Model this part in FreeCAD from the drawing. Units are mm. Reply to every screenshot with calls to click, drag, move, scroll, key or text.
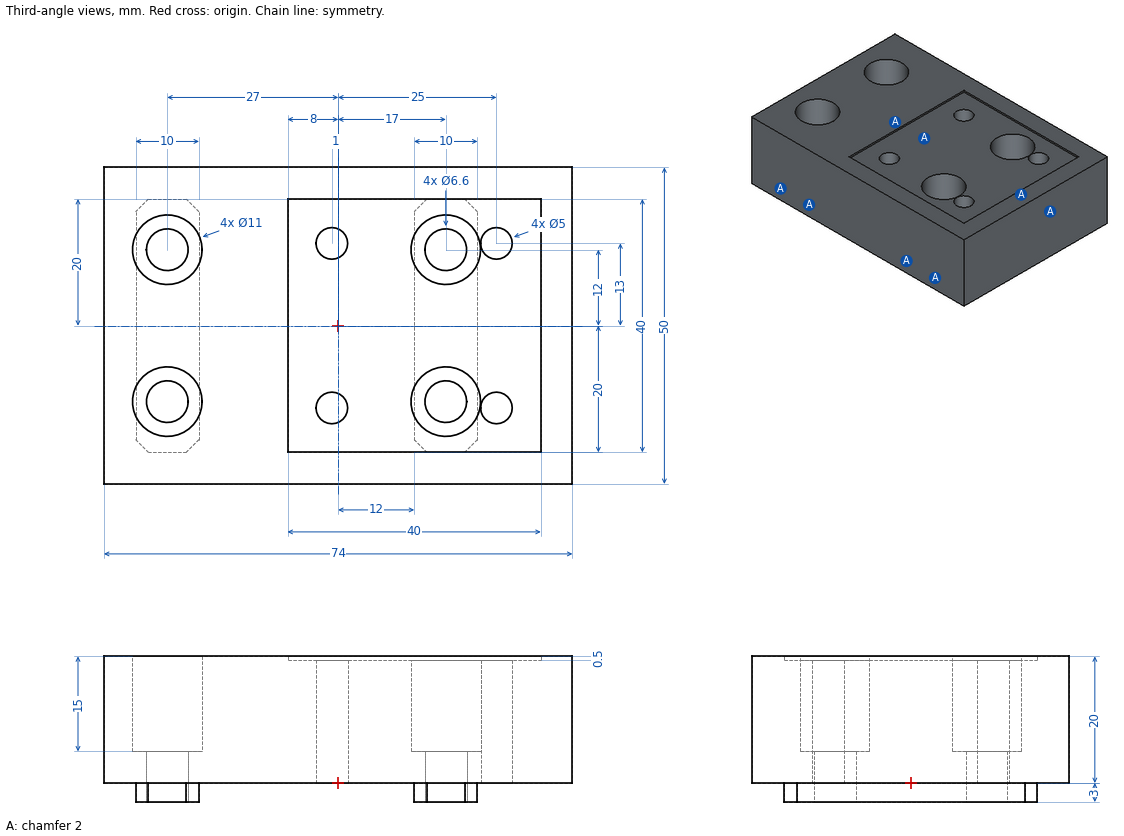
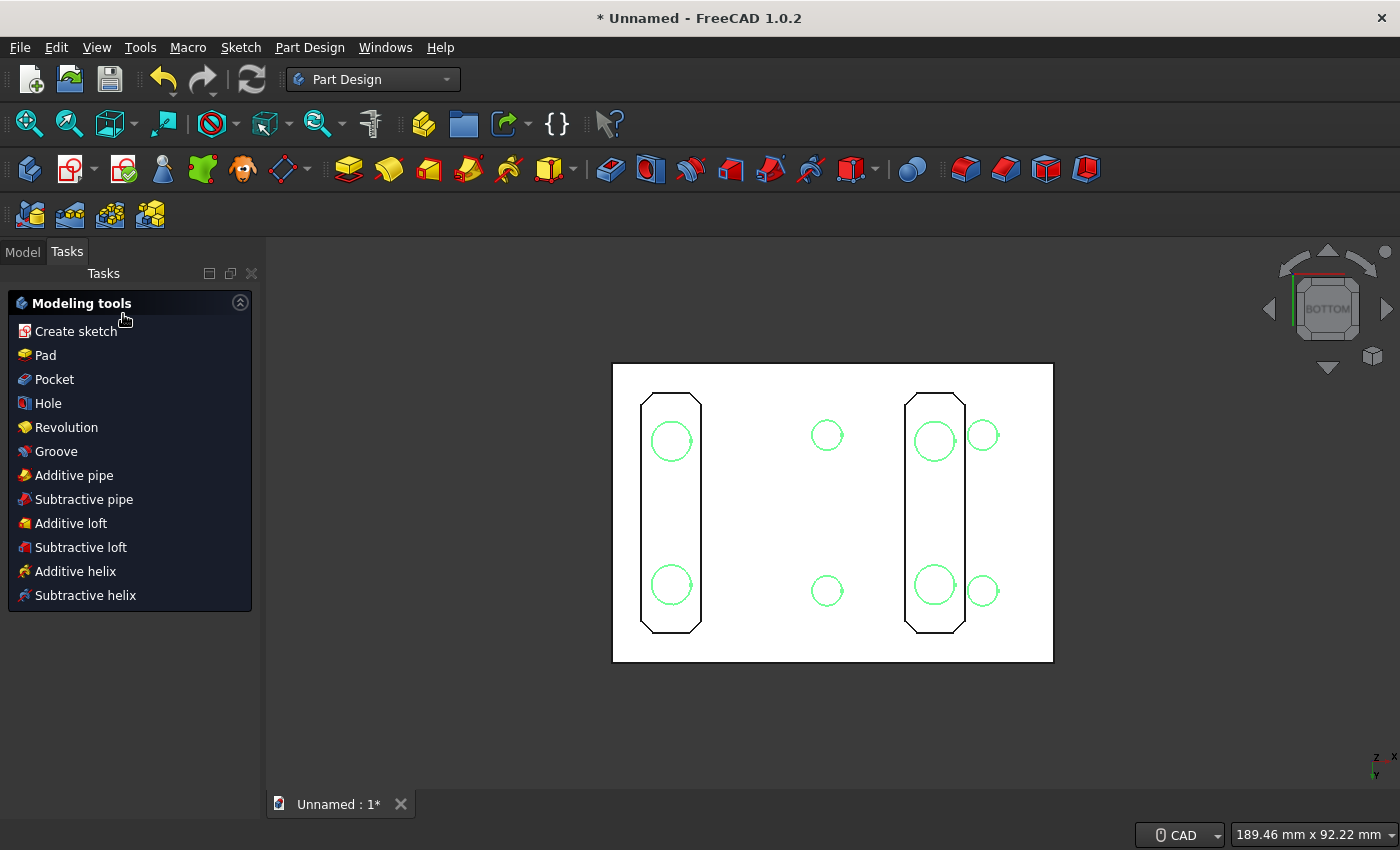
click(612, 170)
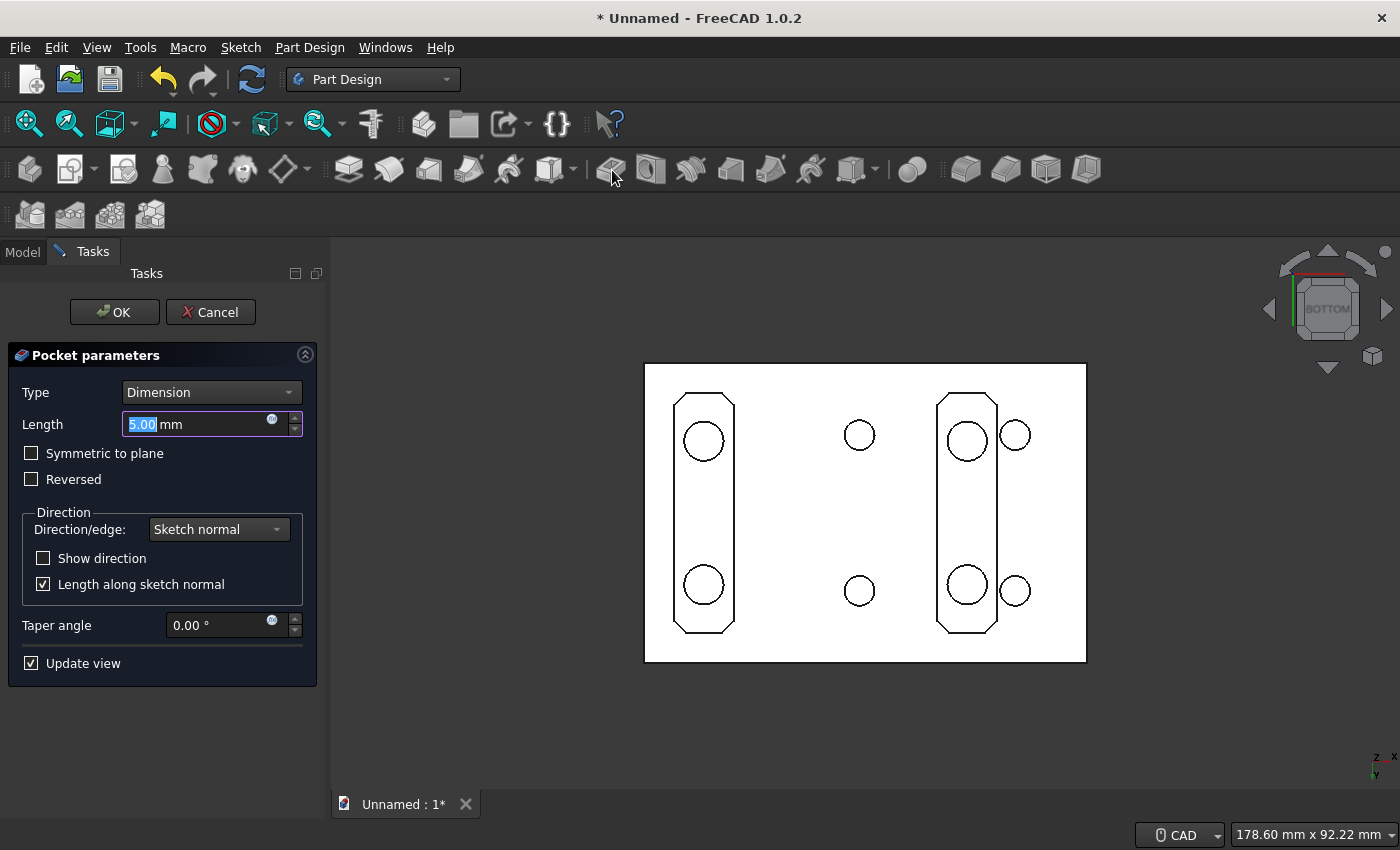
click(212, 392)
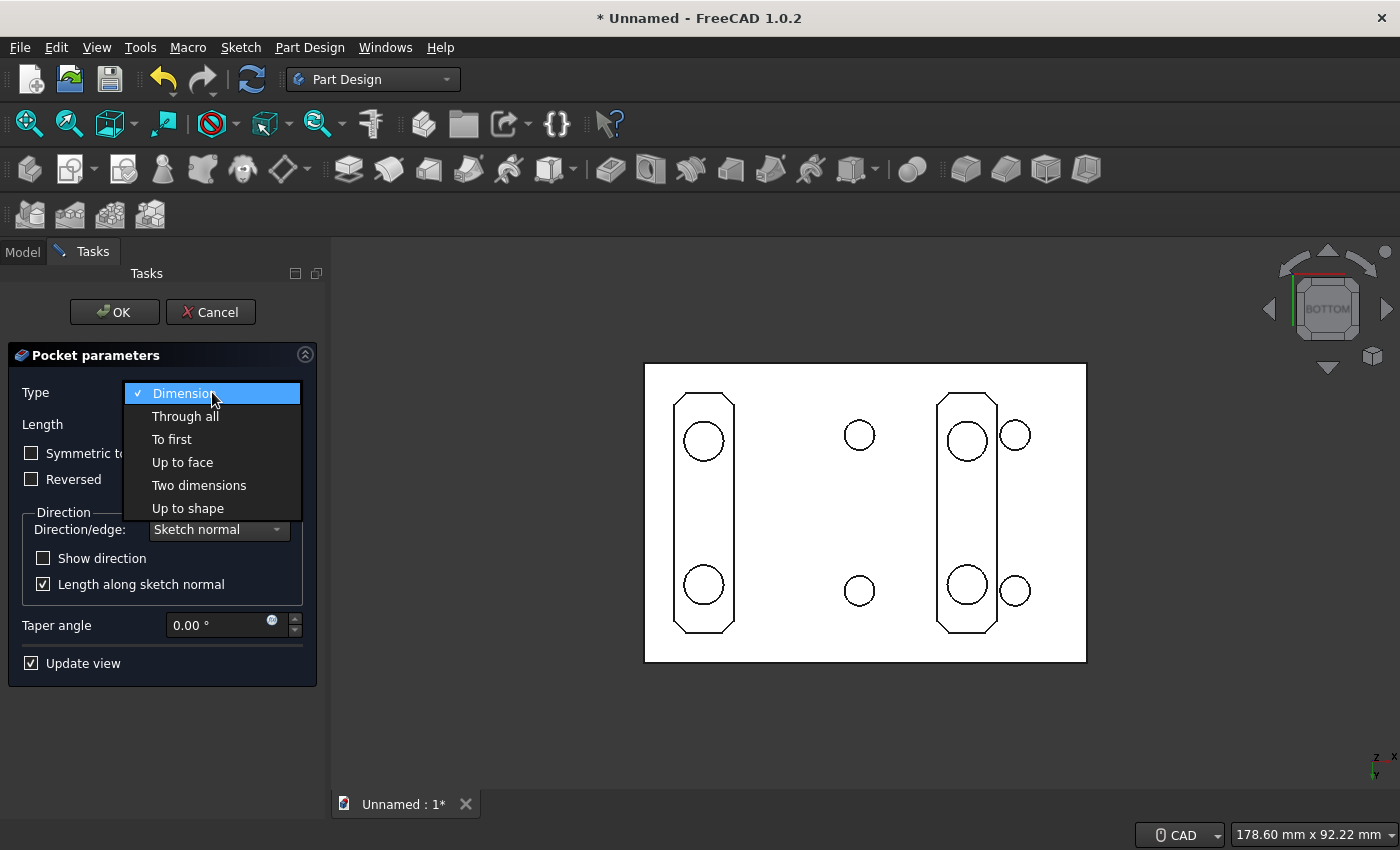
click(212, 416)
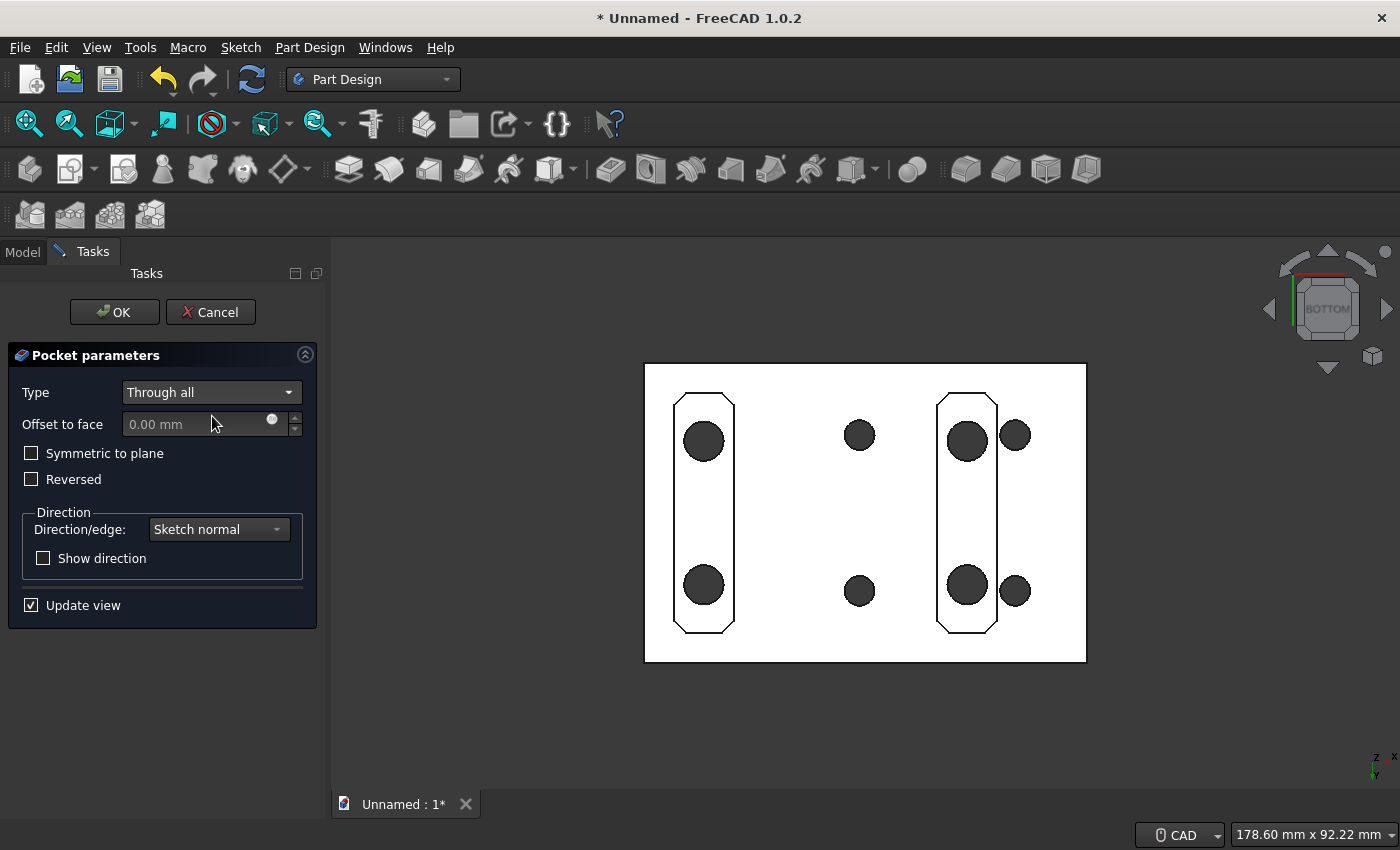
click(115, 312)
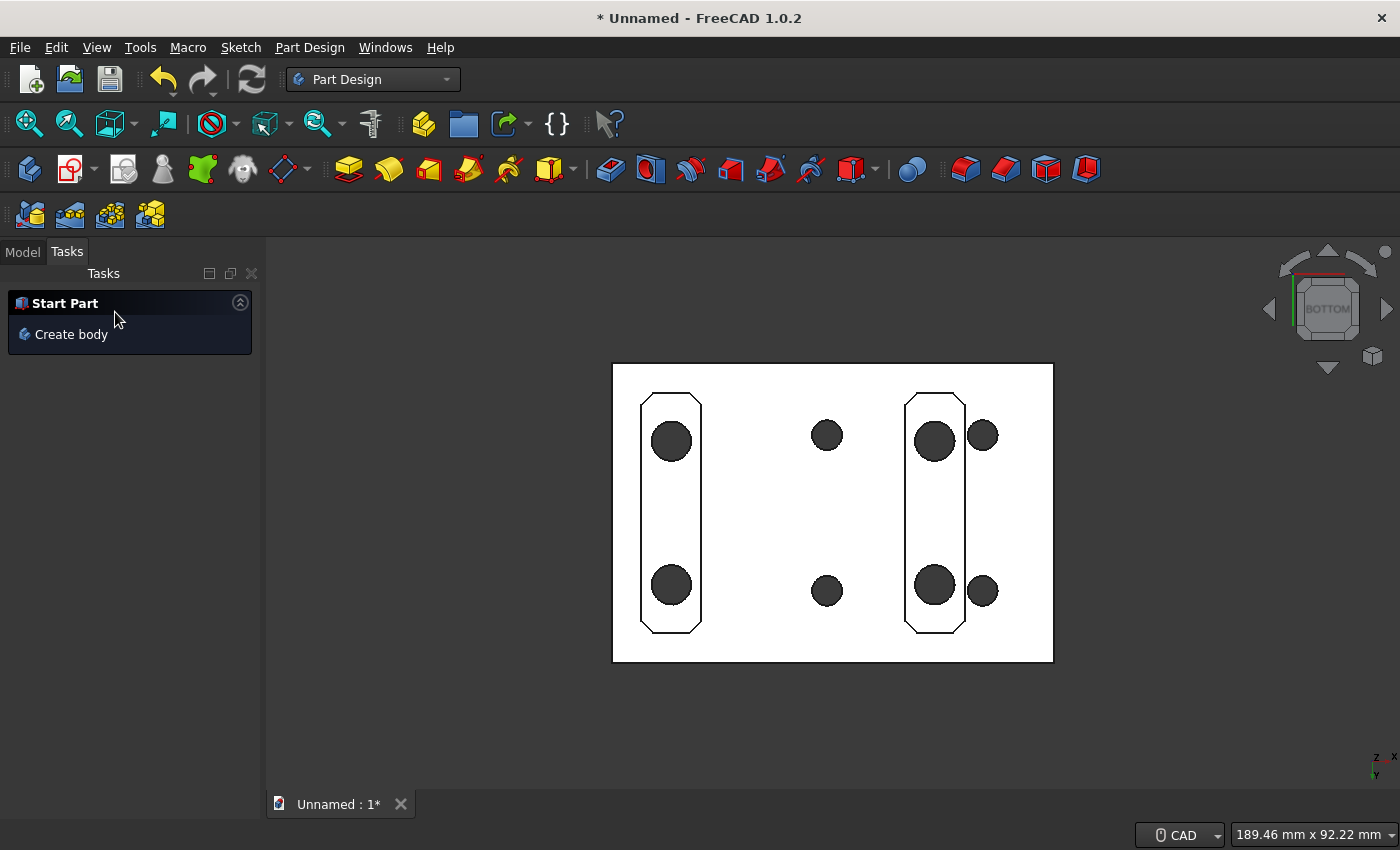
key(0)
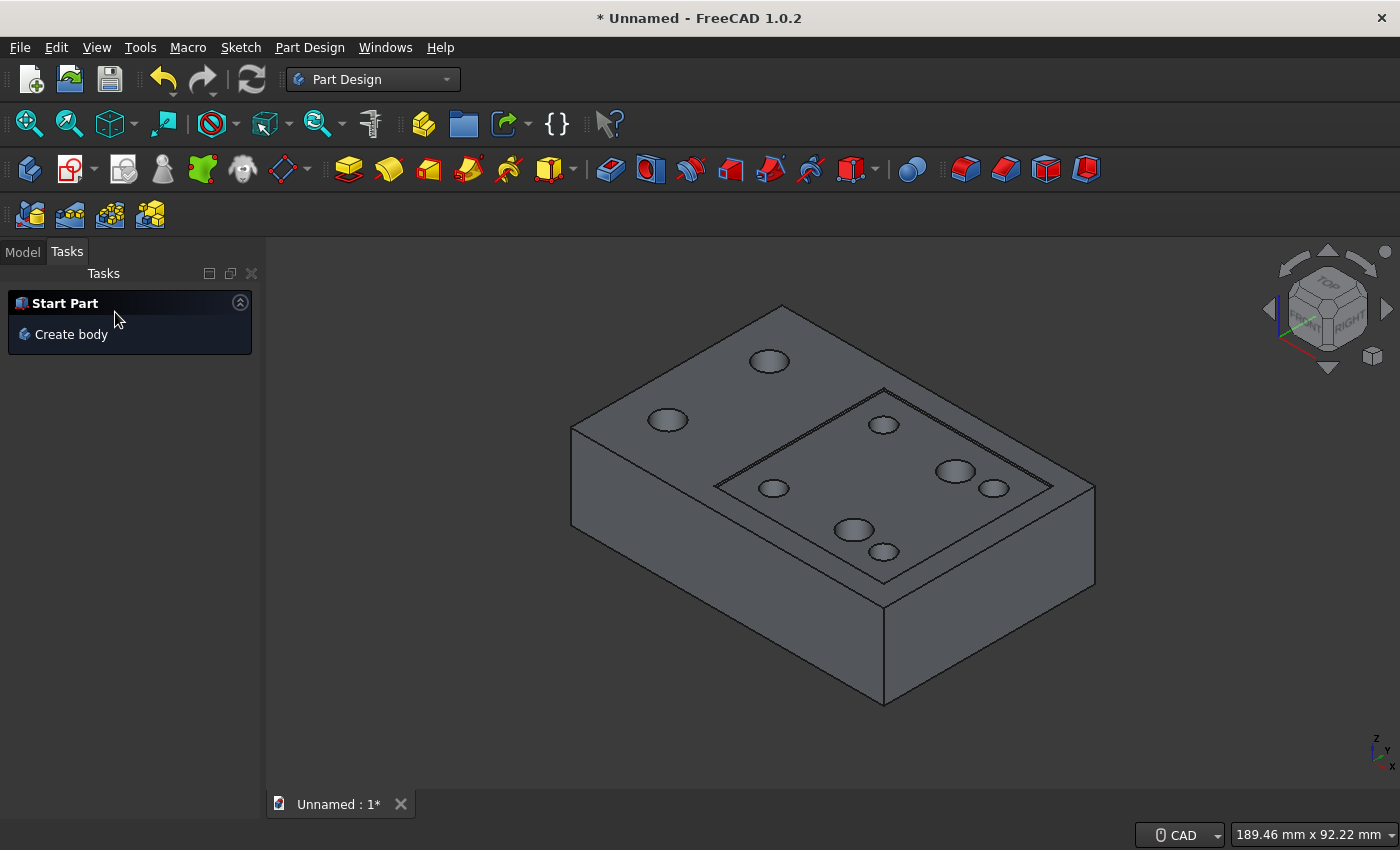
click(744, 404)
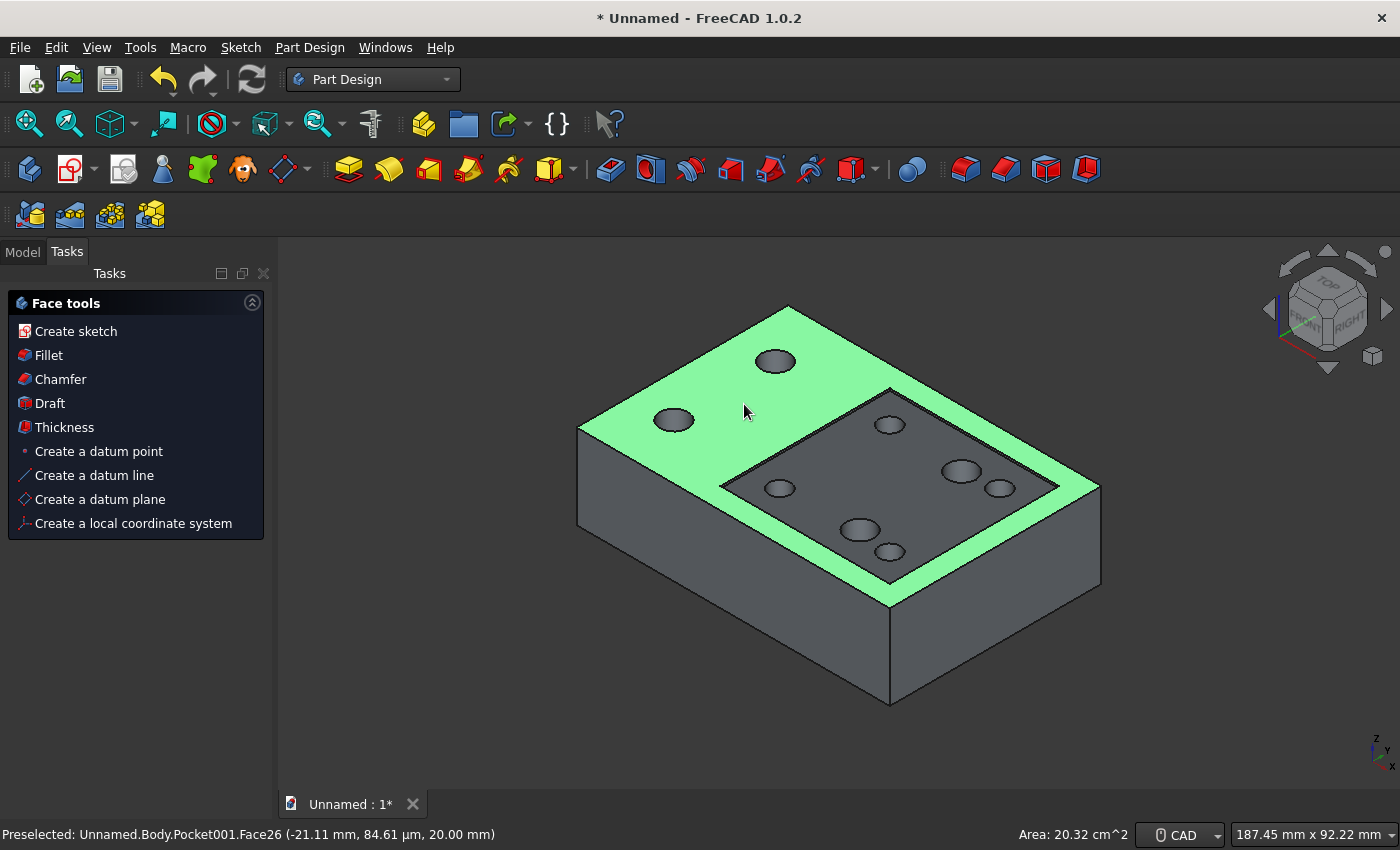
click(70, 170)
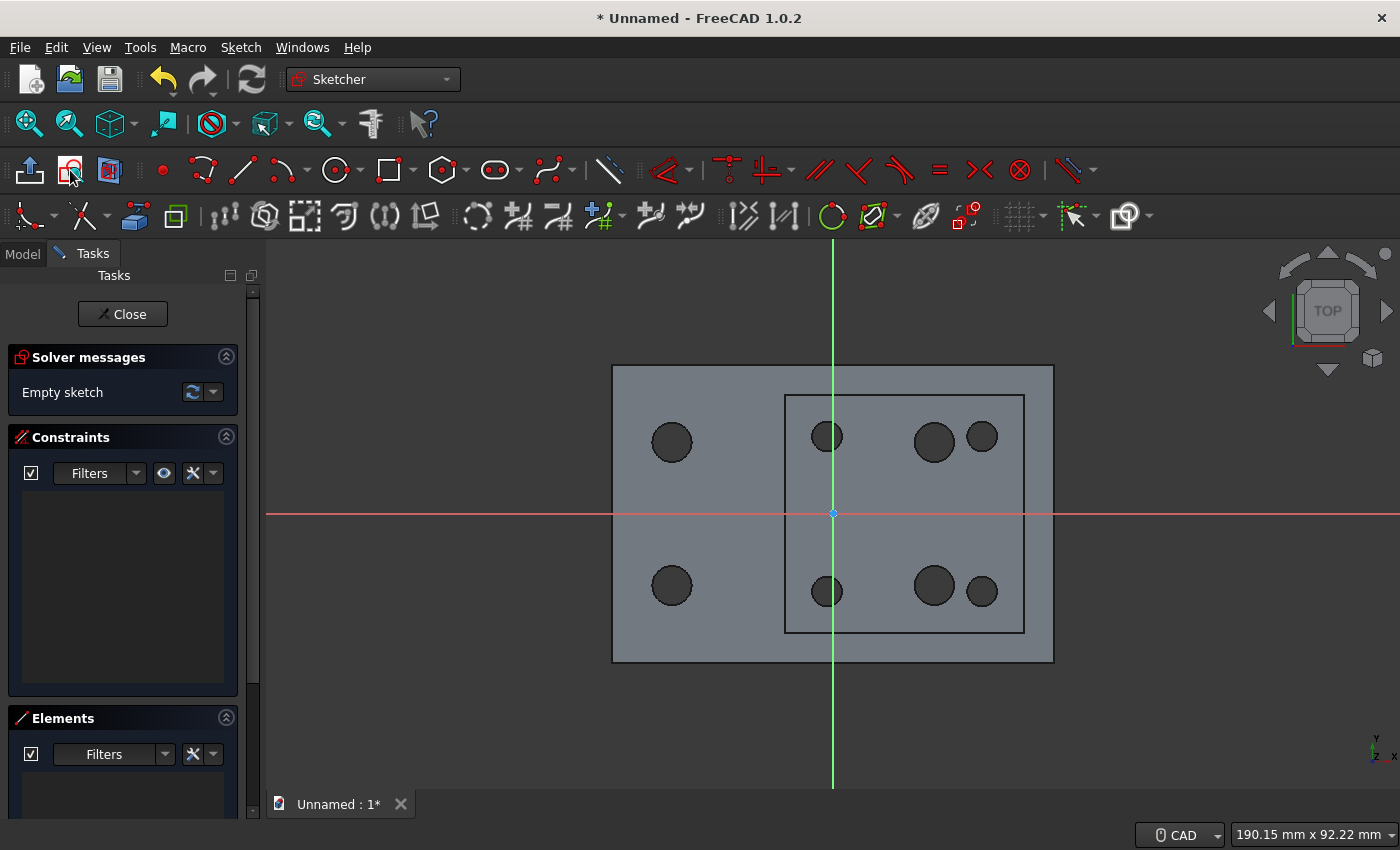
scroll(850, 514, up, 3)